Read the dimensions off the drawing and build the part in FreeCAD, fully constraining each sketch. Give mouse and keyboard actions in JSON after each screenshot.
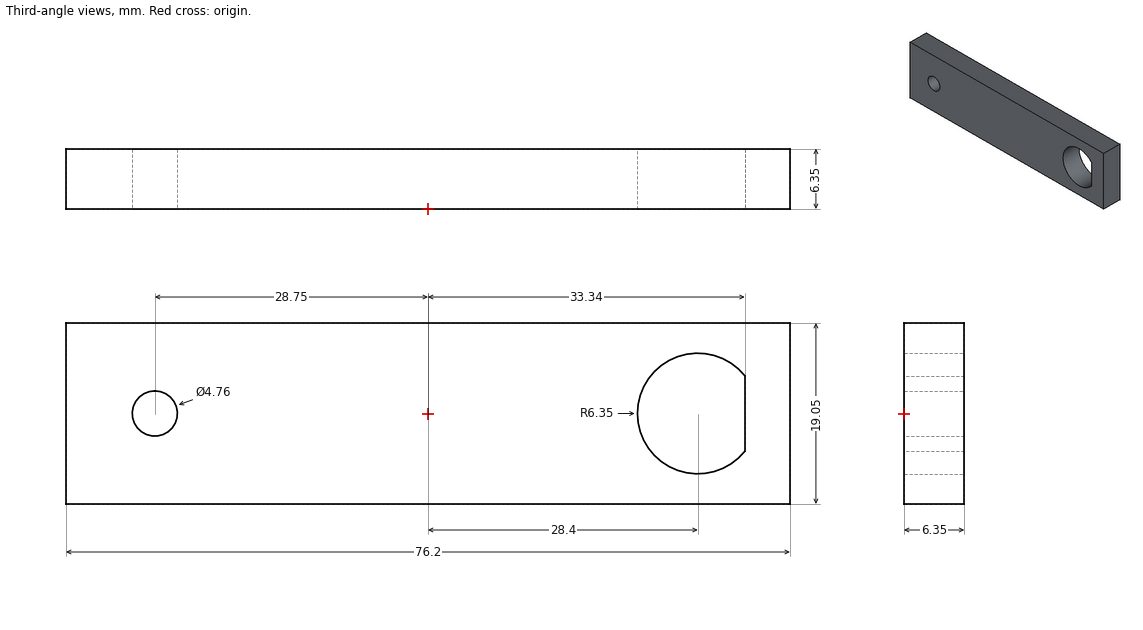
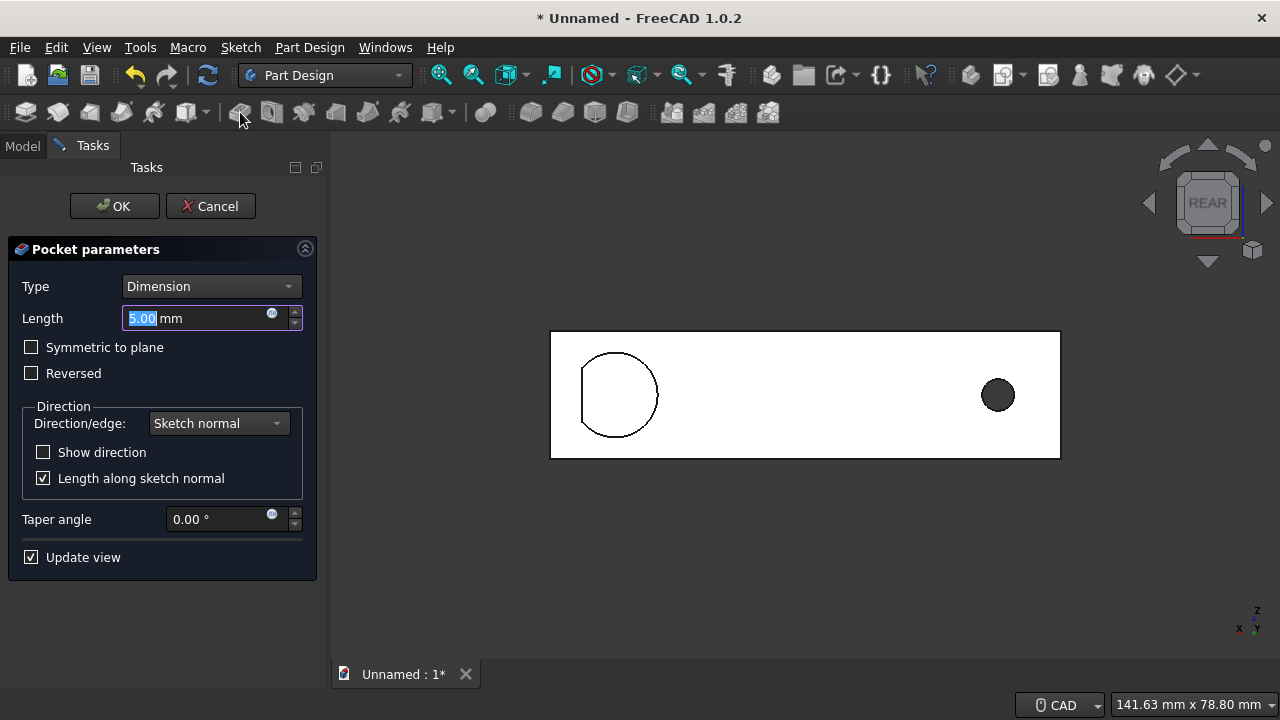
{"action": "type", "text": "6.35"}
{"action": "key", "text": "Tab"}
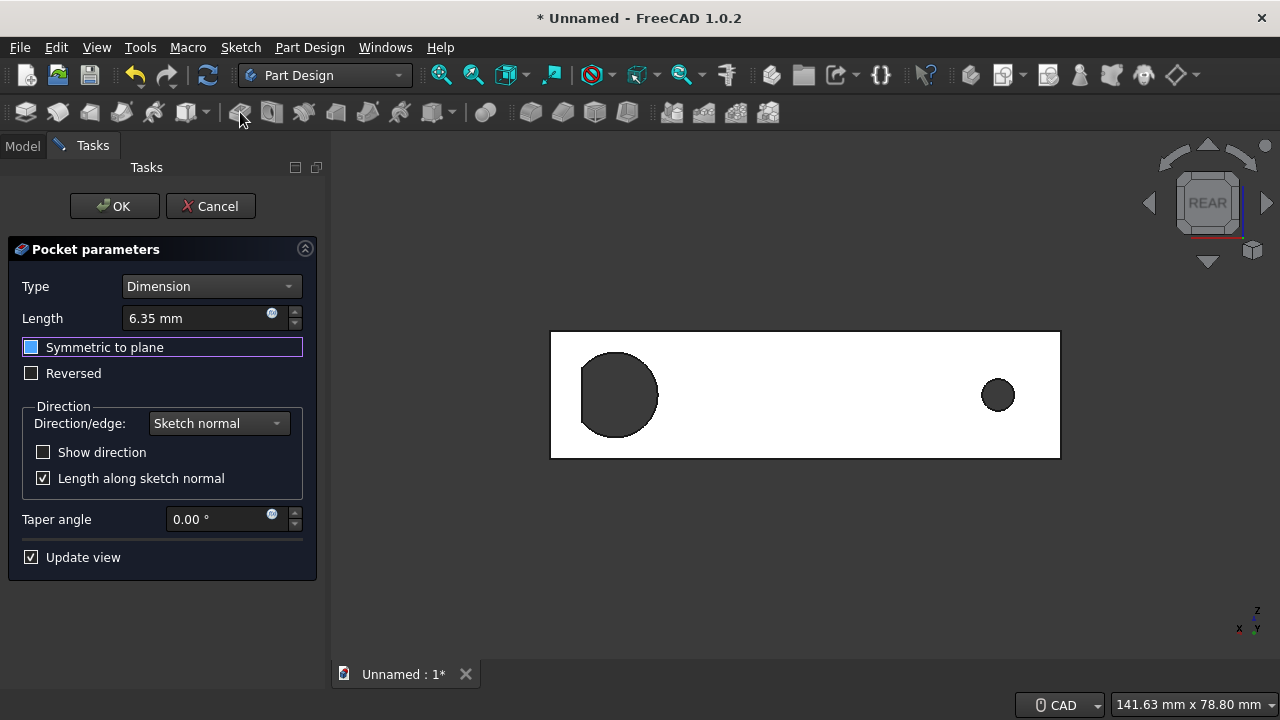
{"action": "left_click", "coordinate": [115, 206]}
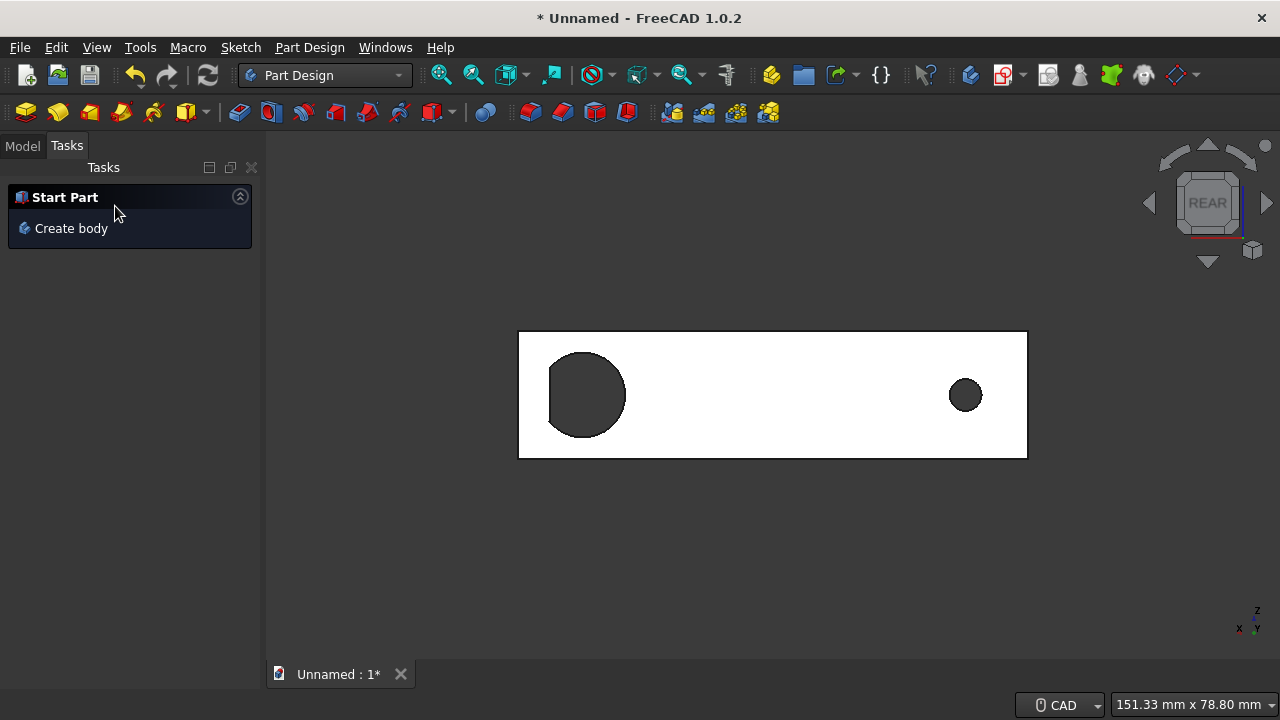
{"action": "key", "text": "0"}